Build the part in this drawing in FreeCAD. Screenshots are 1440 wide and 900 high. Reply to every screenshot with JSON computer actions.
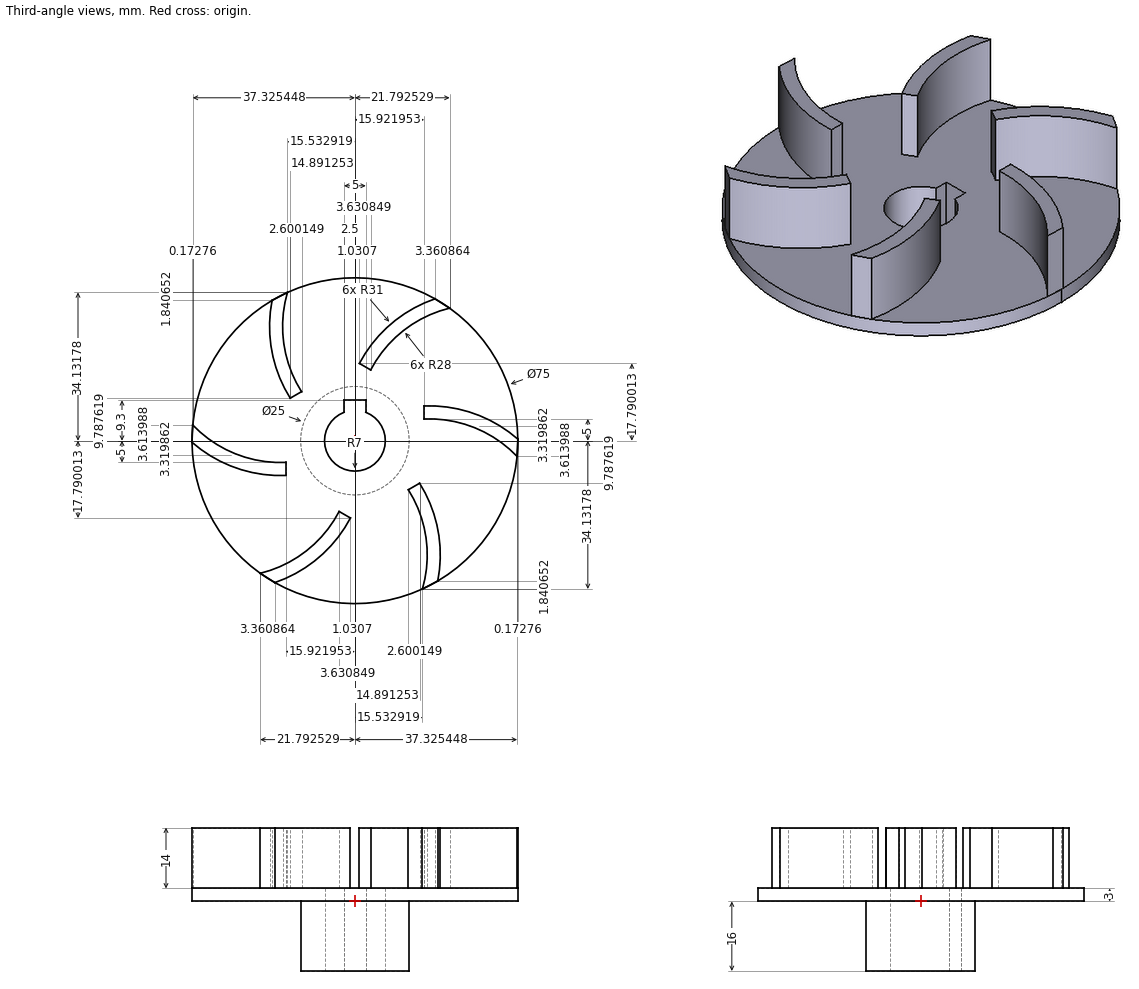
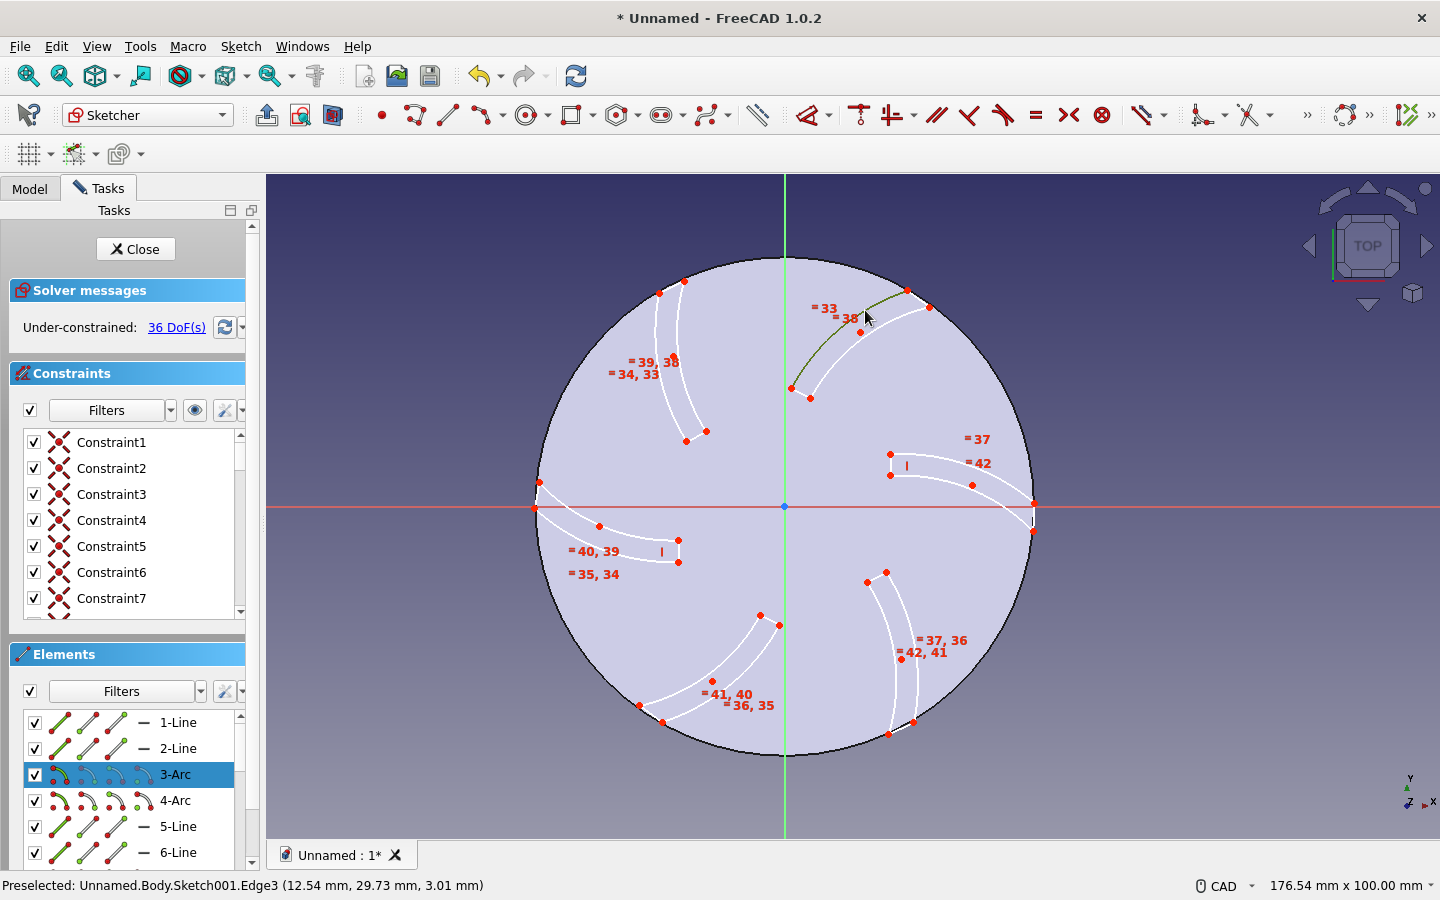
{"action": "key", "text": "k r"}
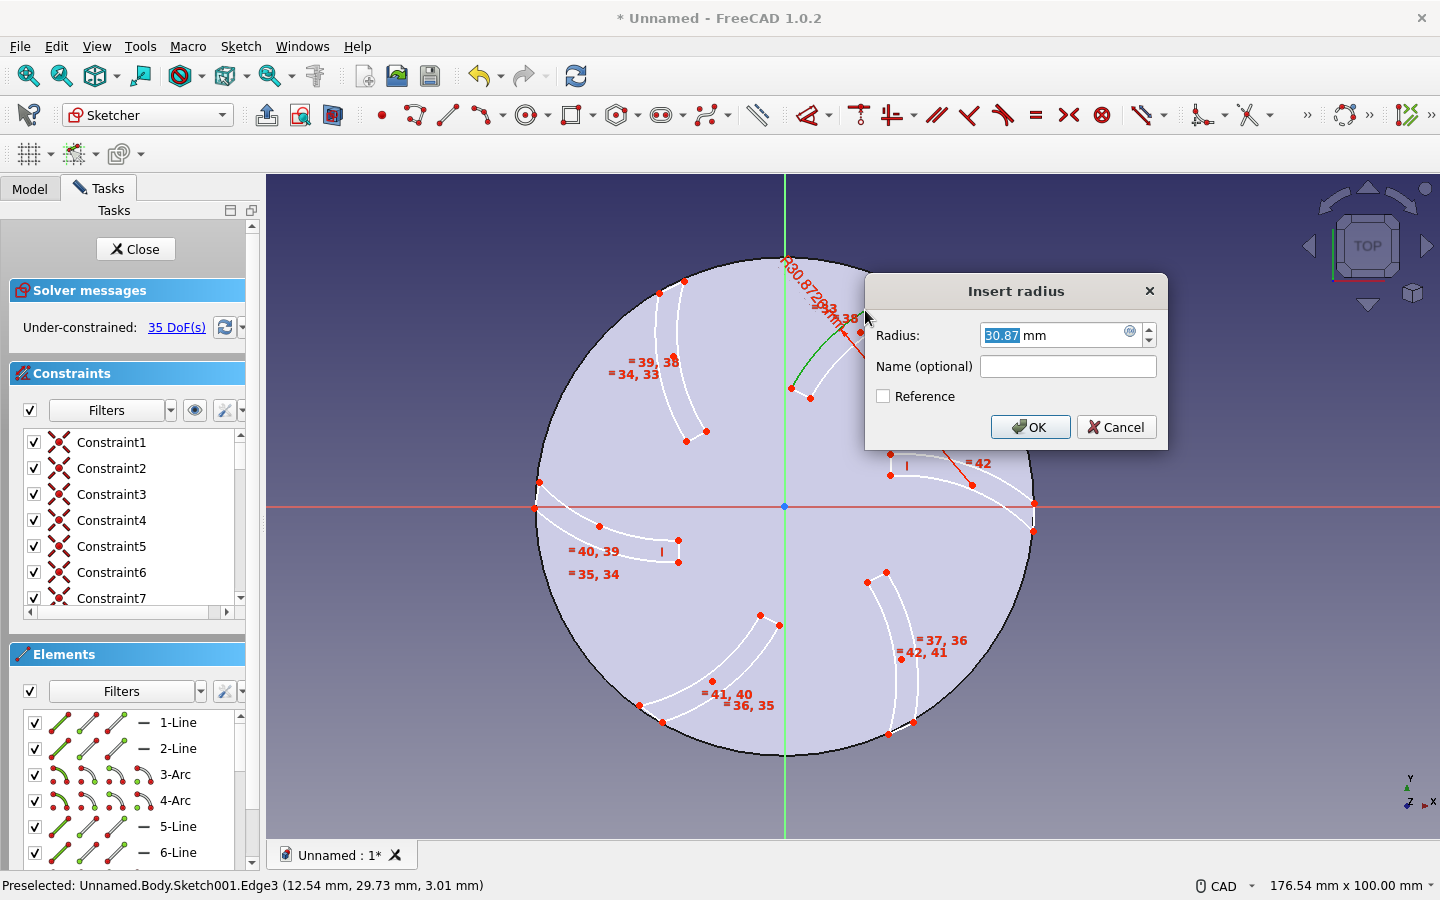
{"action": "type", "text": "31"}
{"action": "key", "text": "Return"}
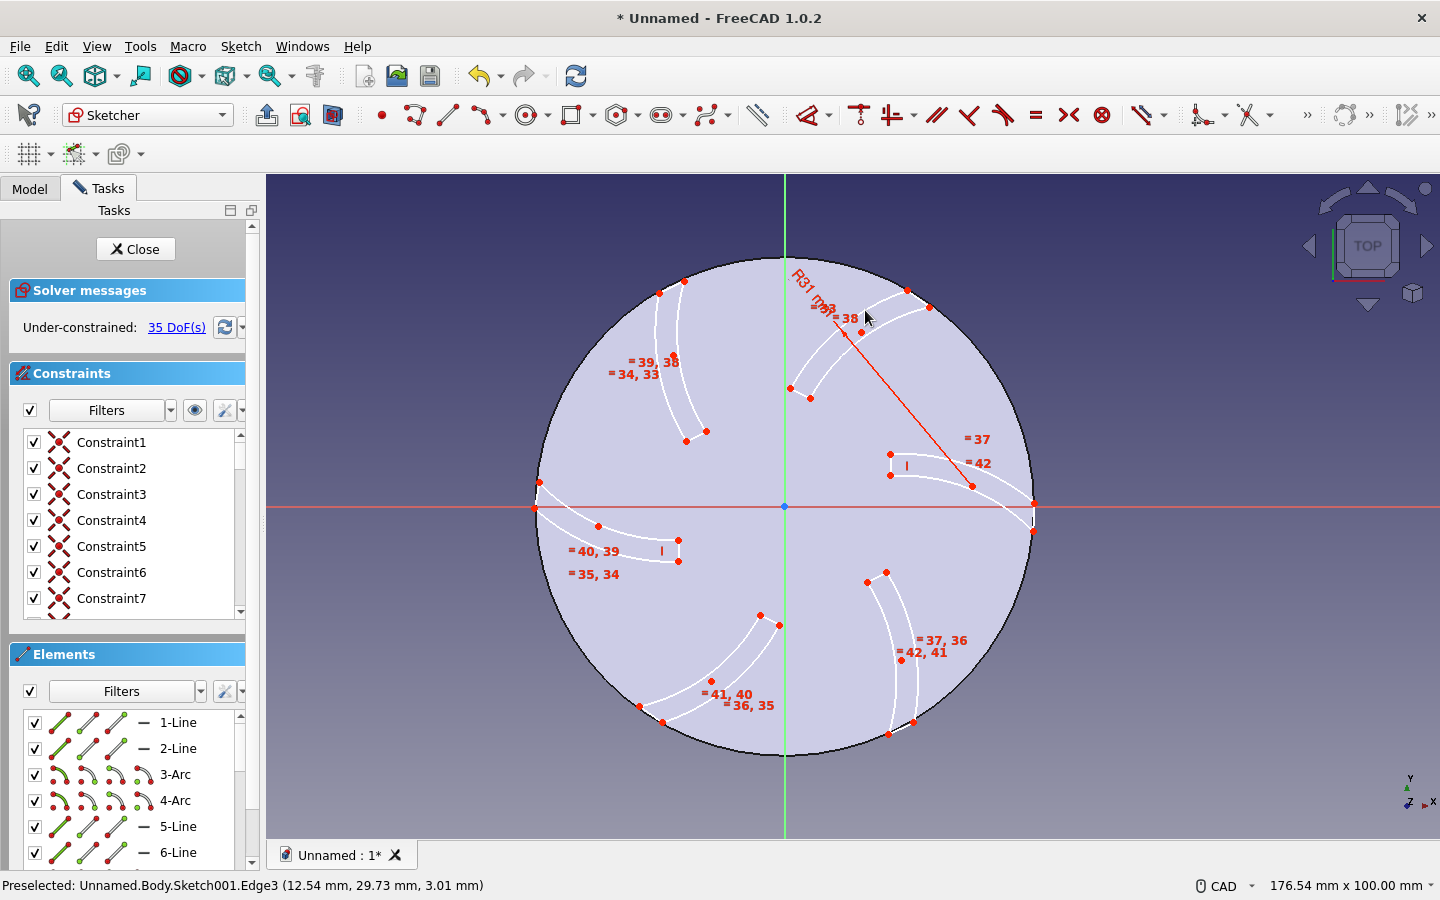
{"action": "left_click", "coordinate": [886, 323]}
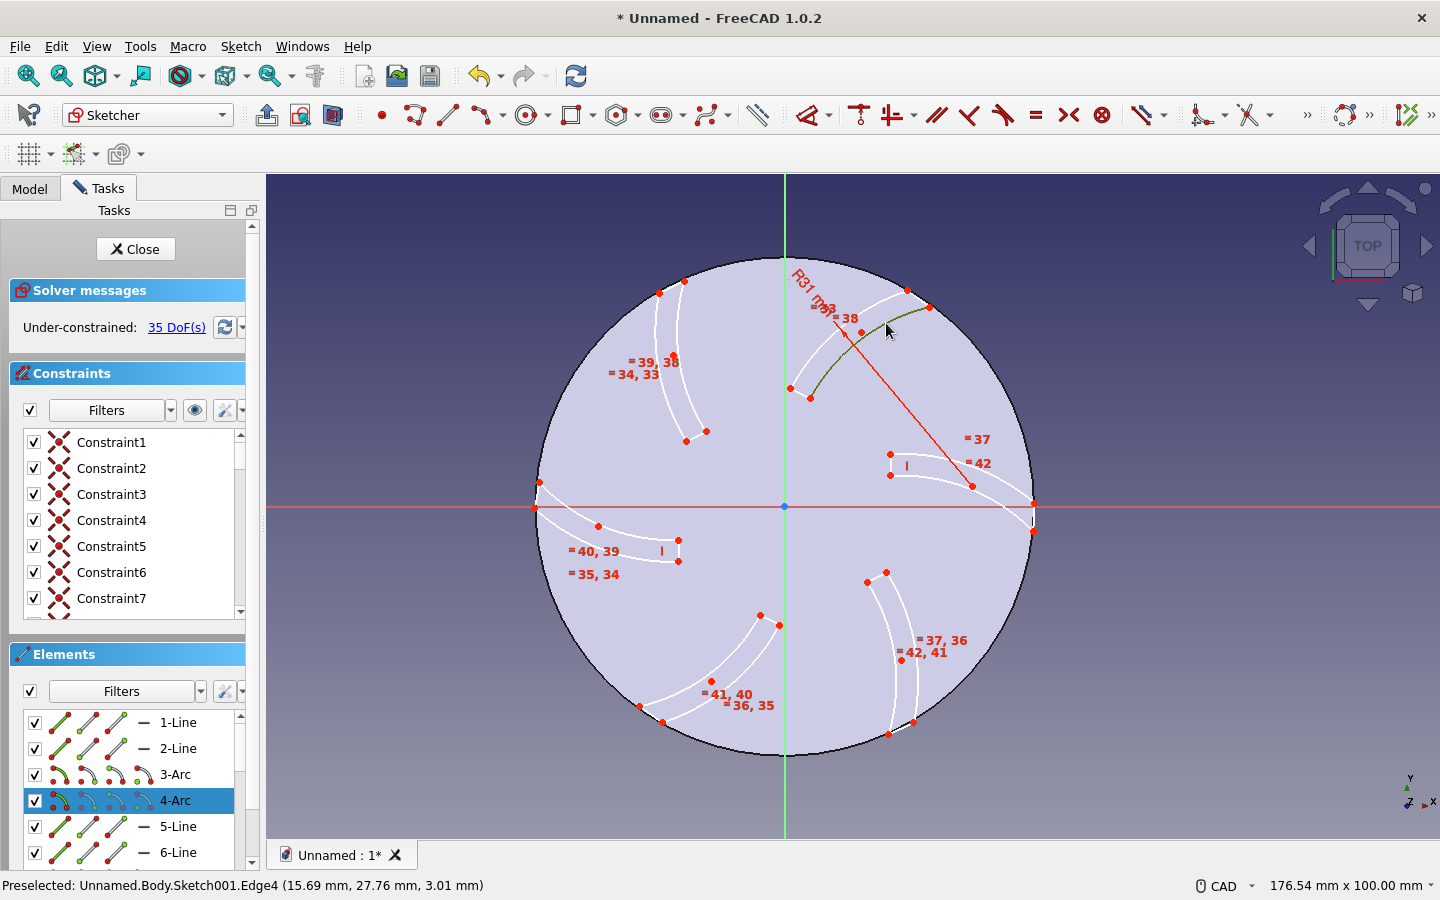
{"action": "key", "text": "k r"}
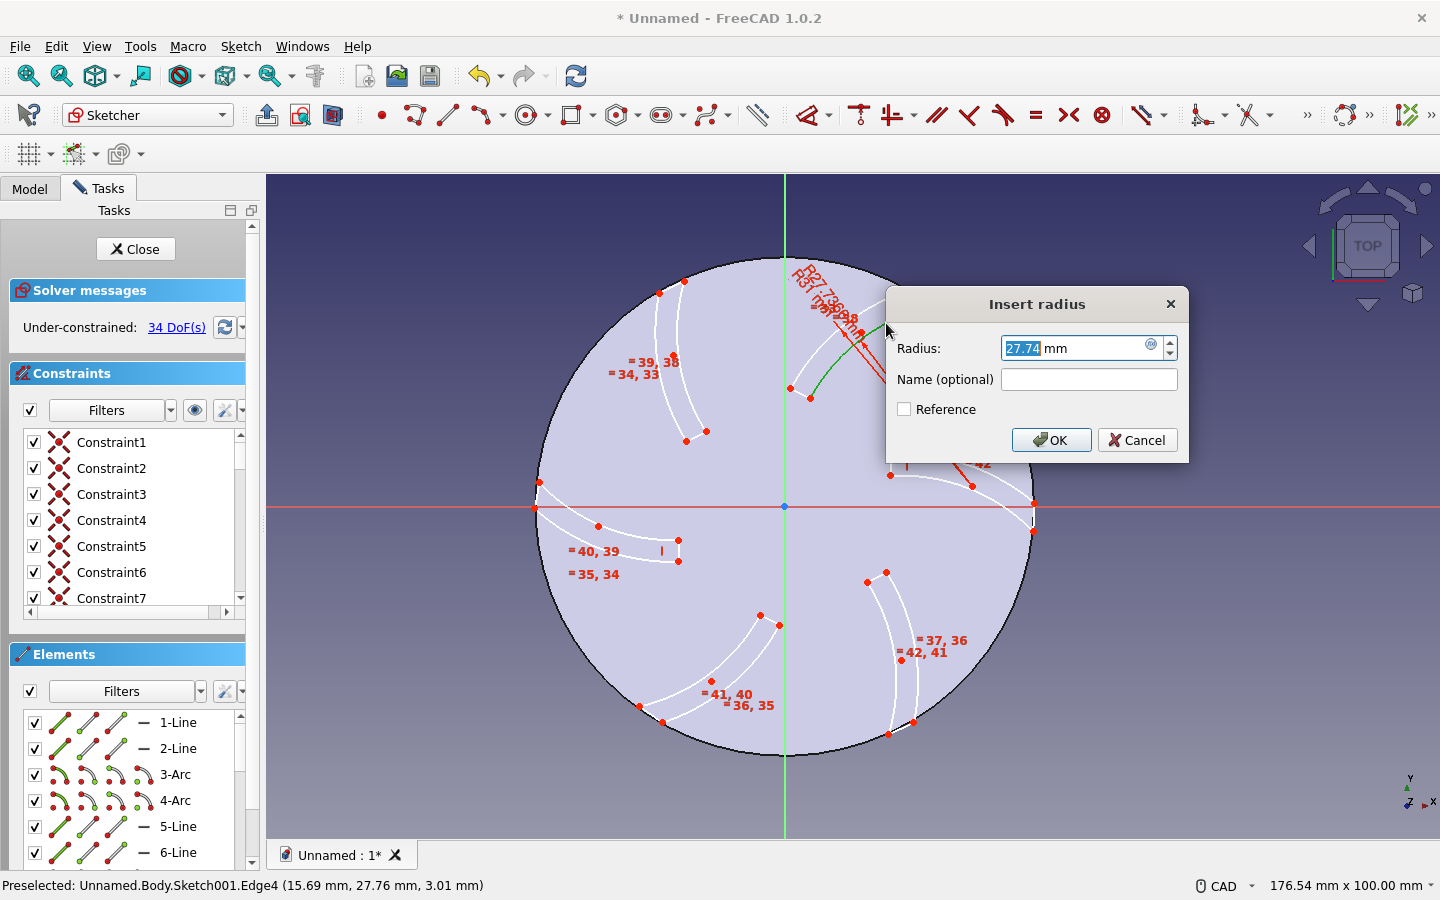
{"action": "type", "text": "28"}
{"action": "key", "text": "Return"}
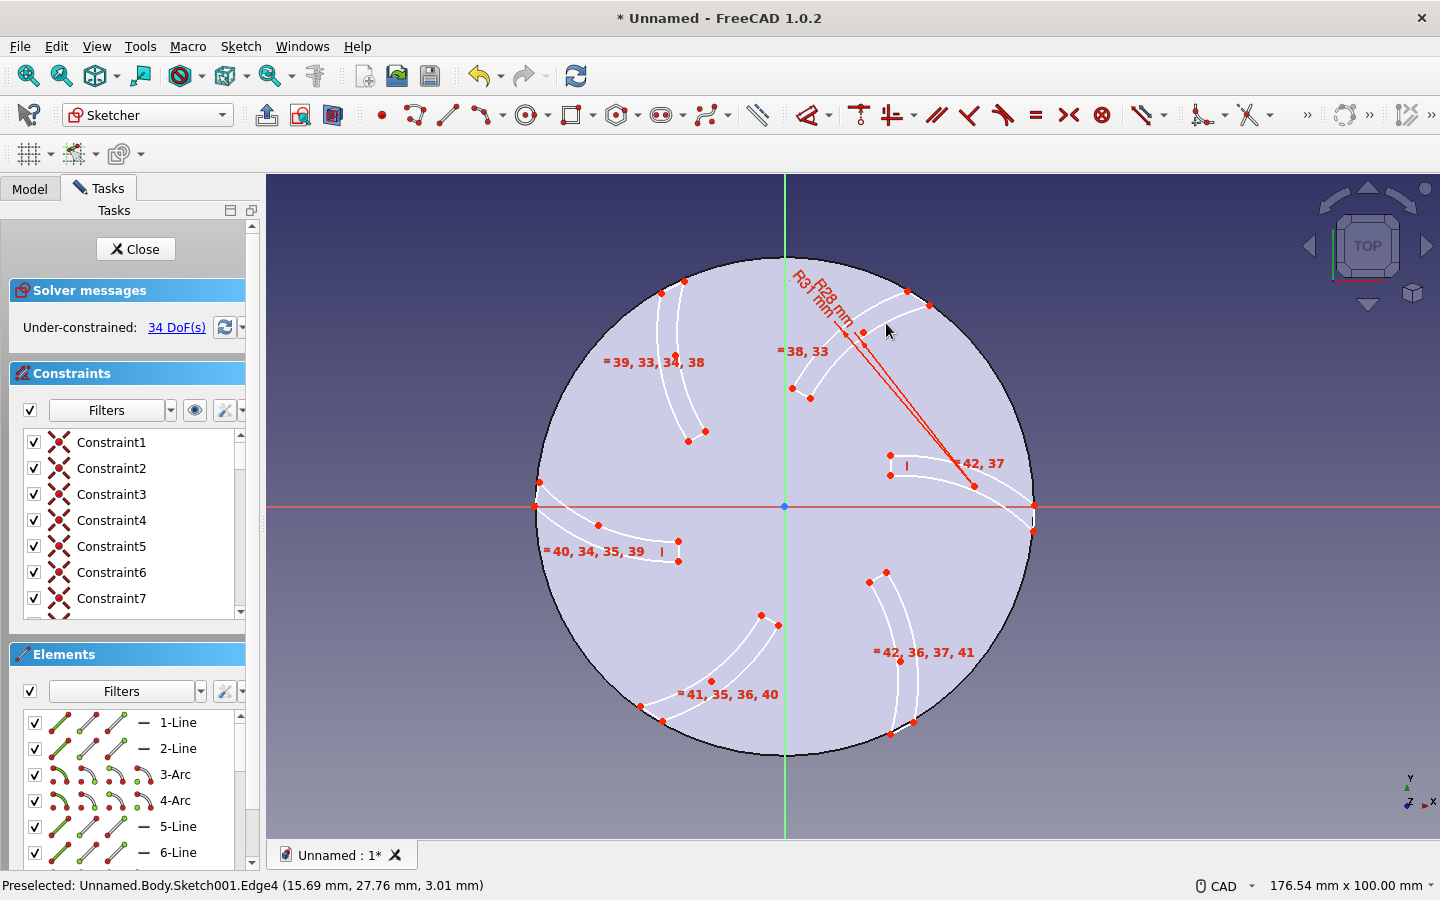
{"action": "left_click", "coordinate": [679, 542]}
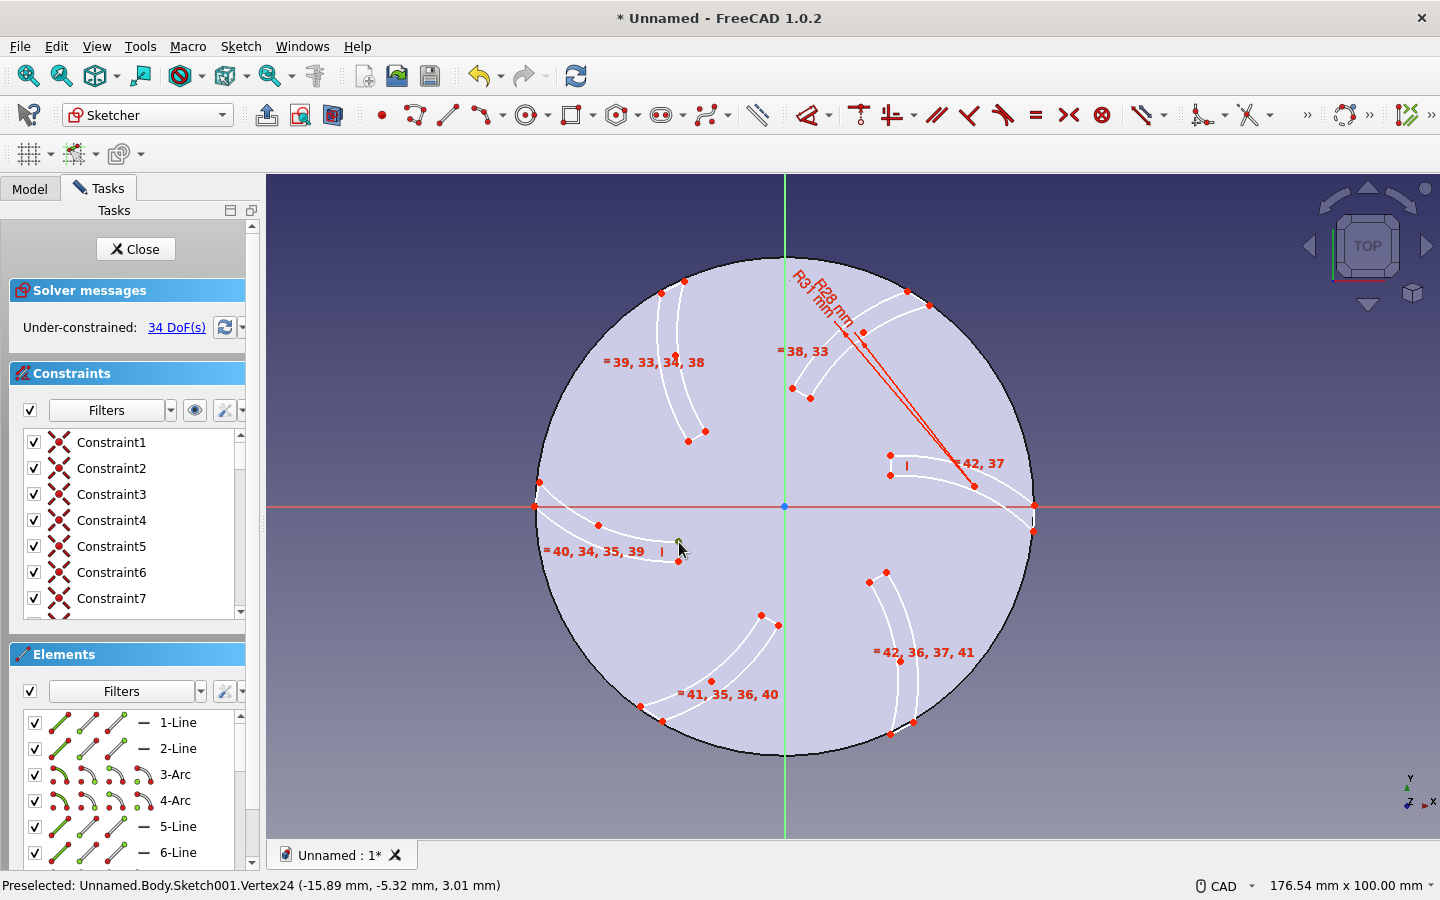
{"action": "key", "text": "i"}